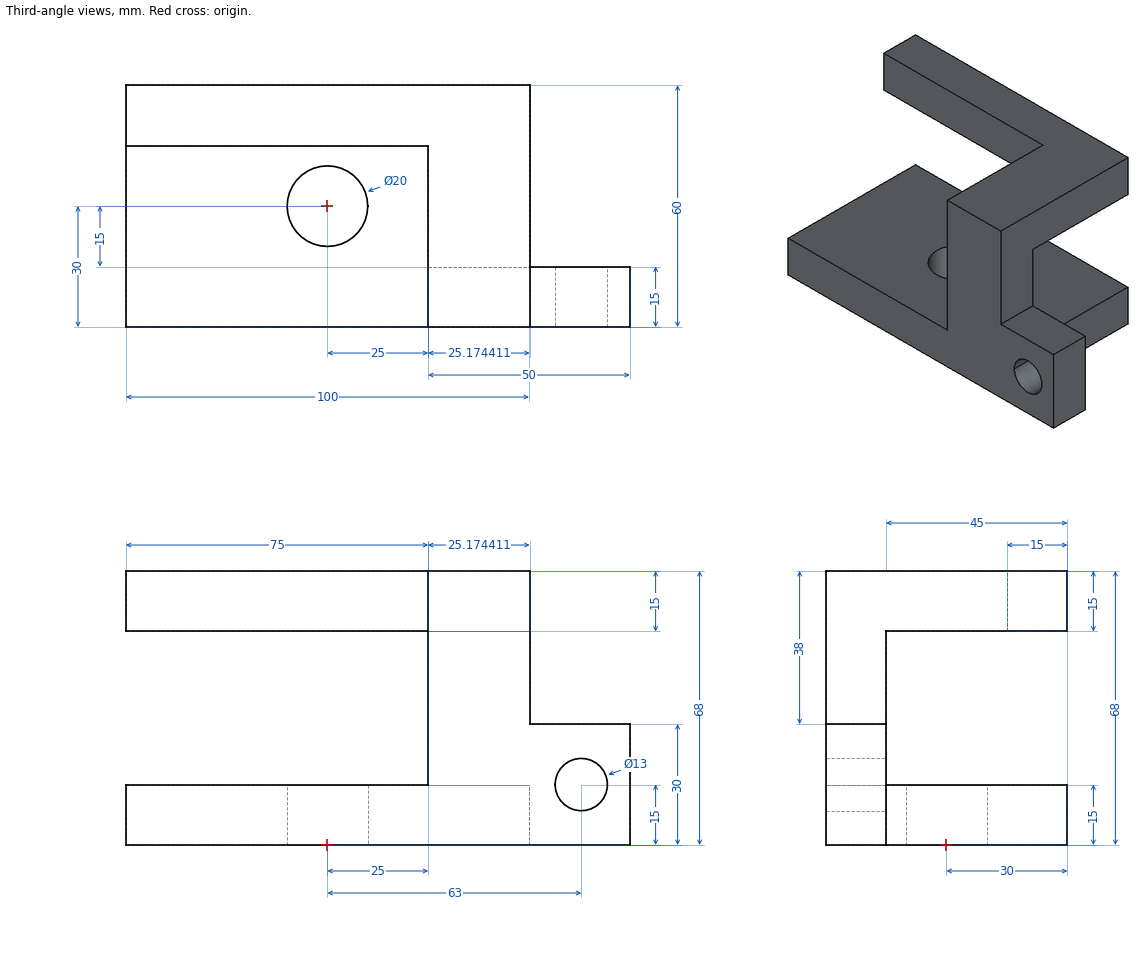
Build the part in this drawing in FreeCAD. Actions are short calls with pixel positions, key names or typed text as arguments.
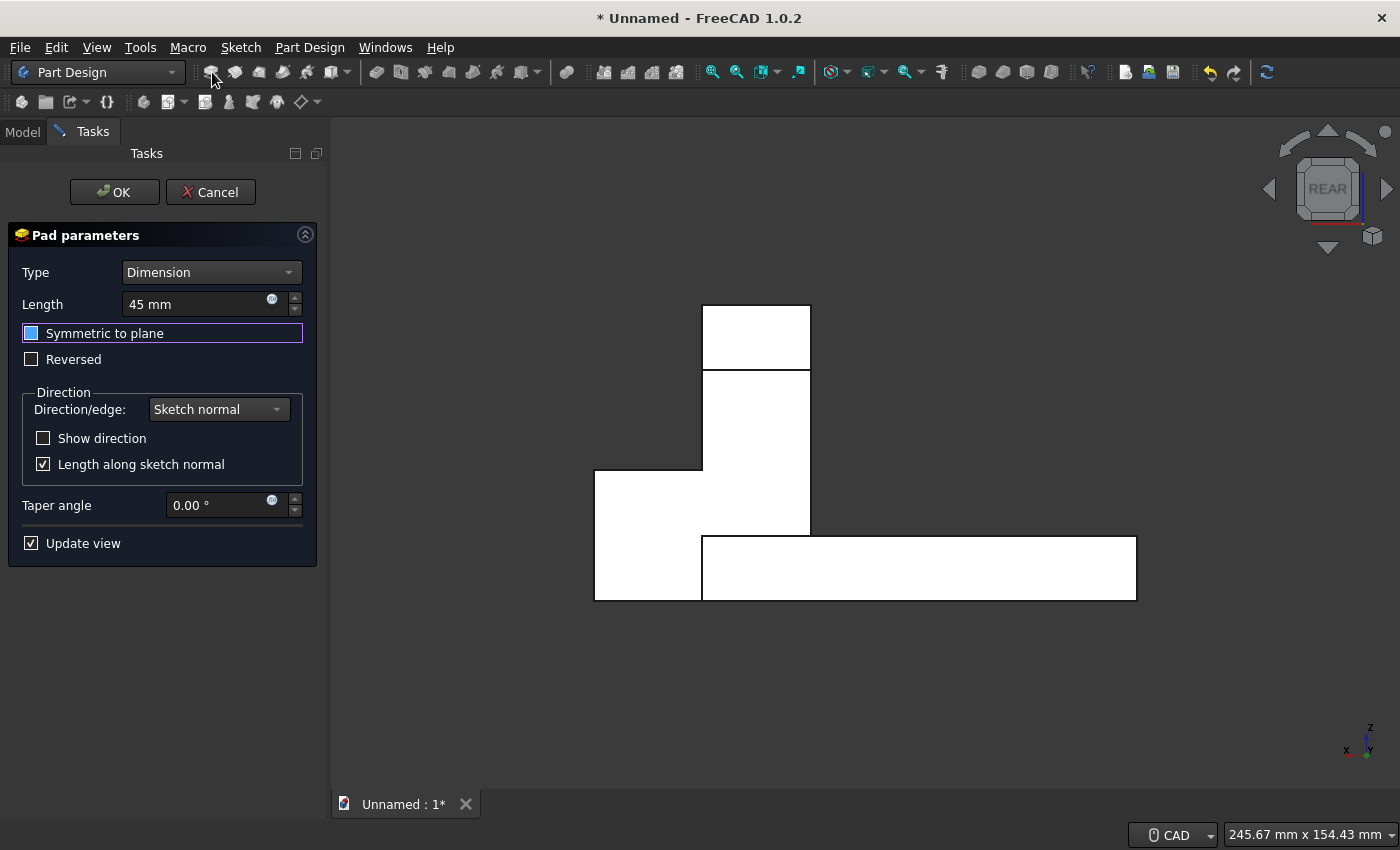
click(115, 192)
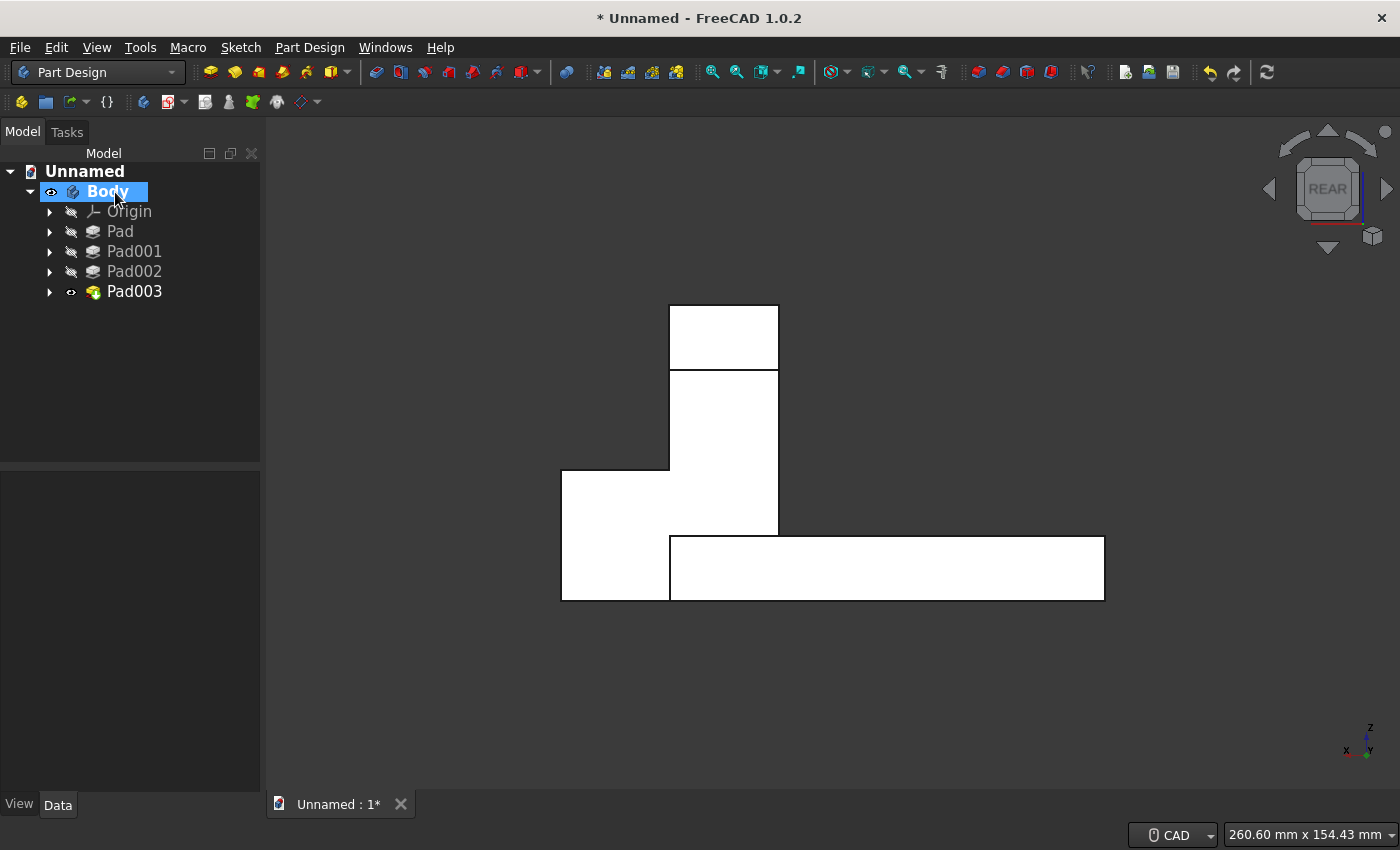
key(6)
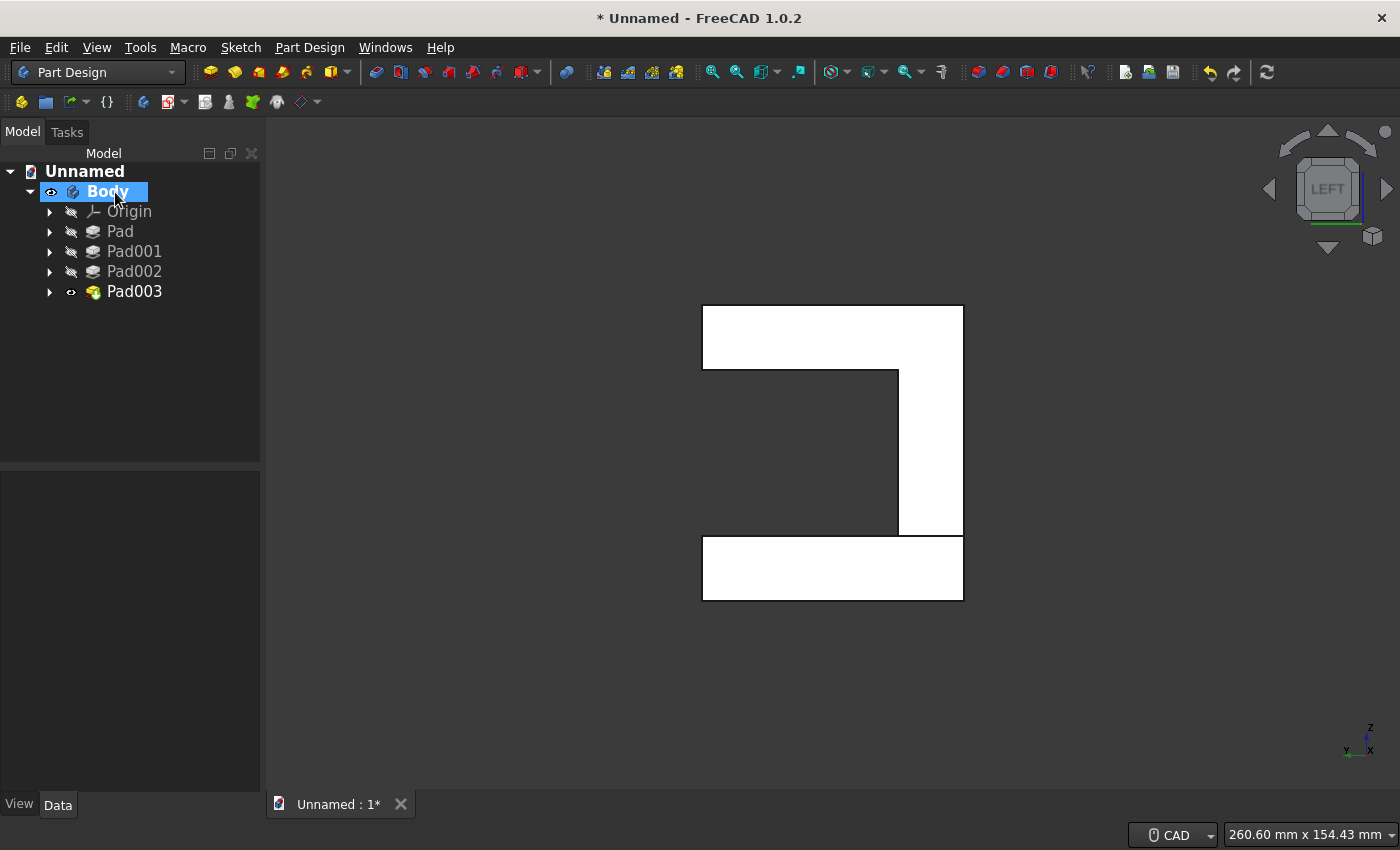
key(v)
key(f)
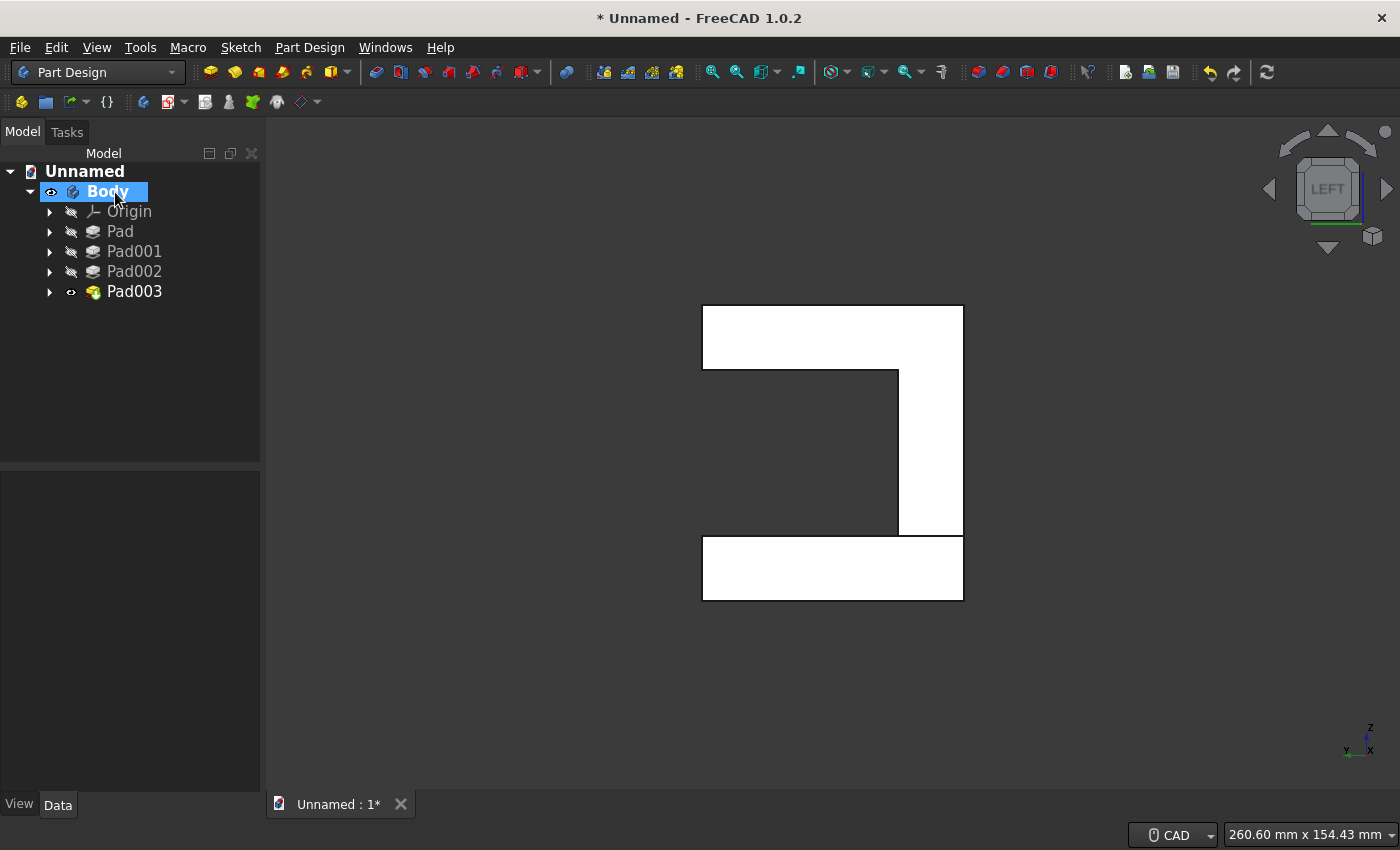
click(945, 353)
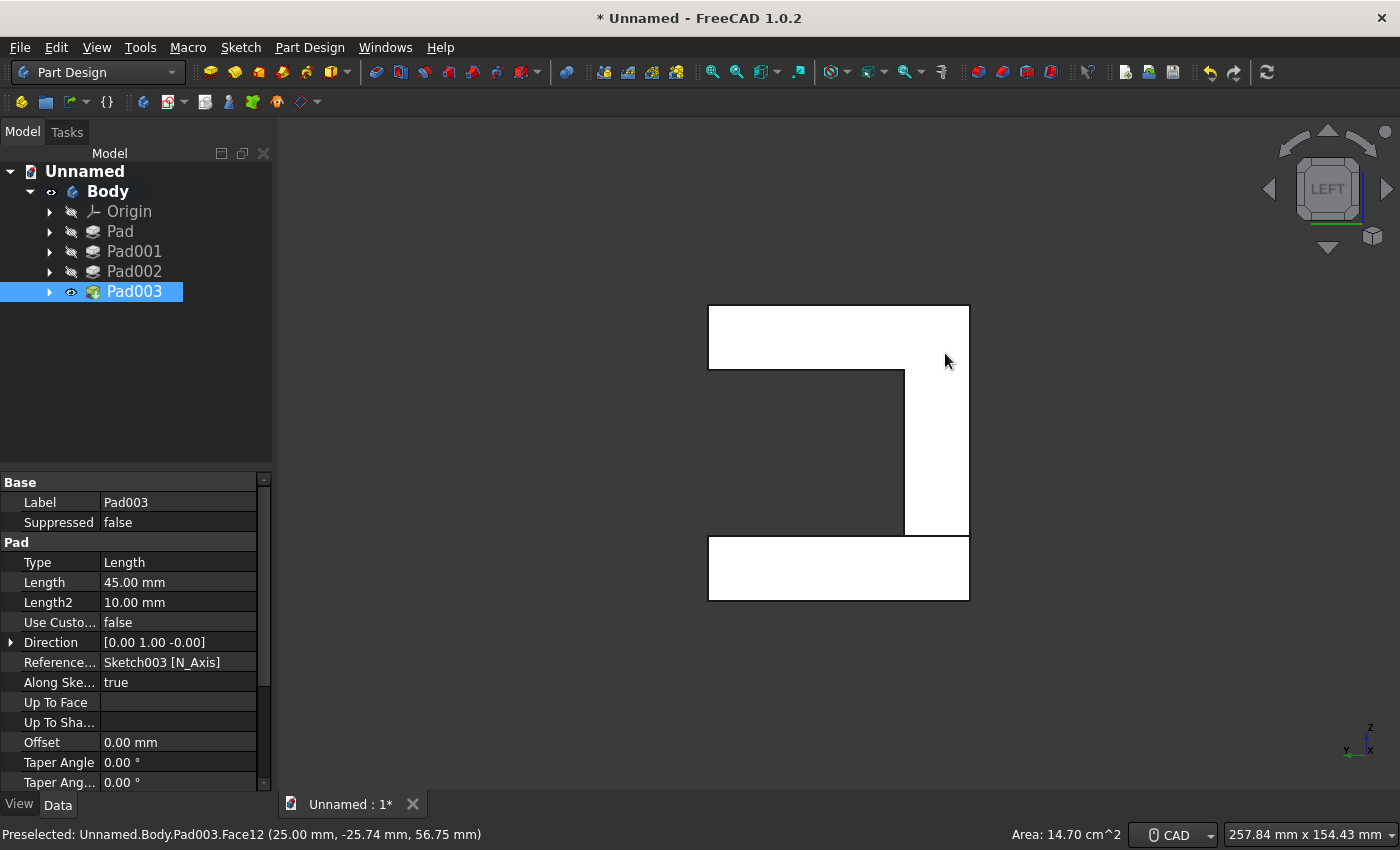
click(168, 102)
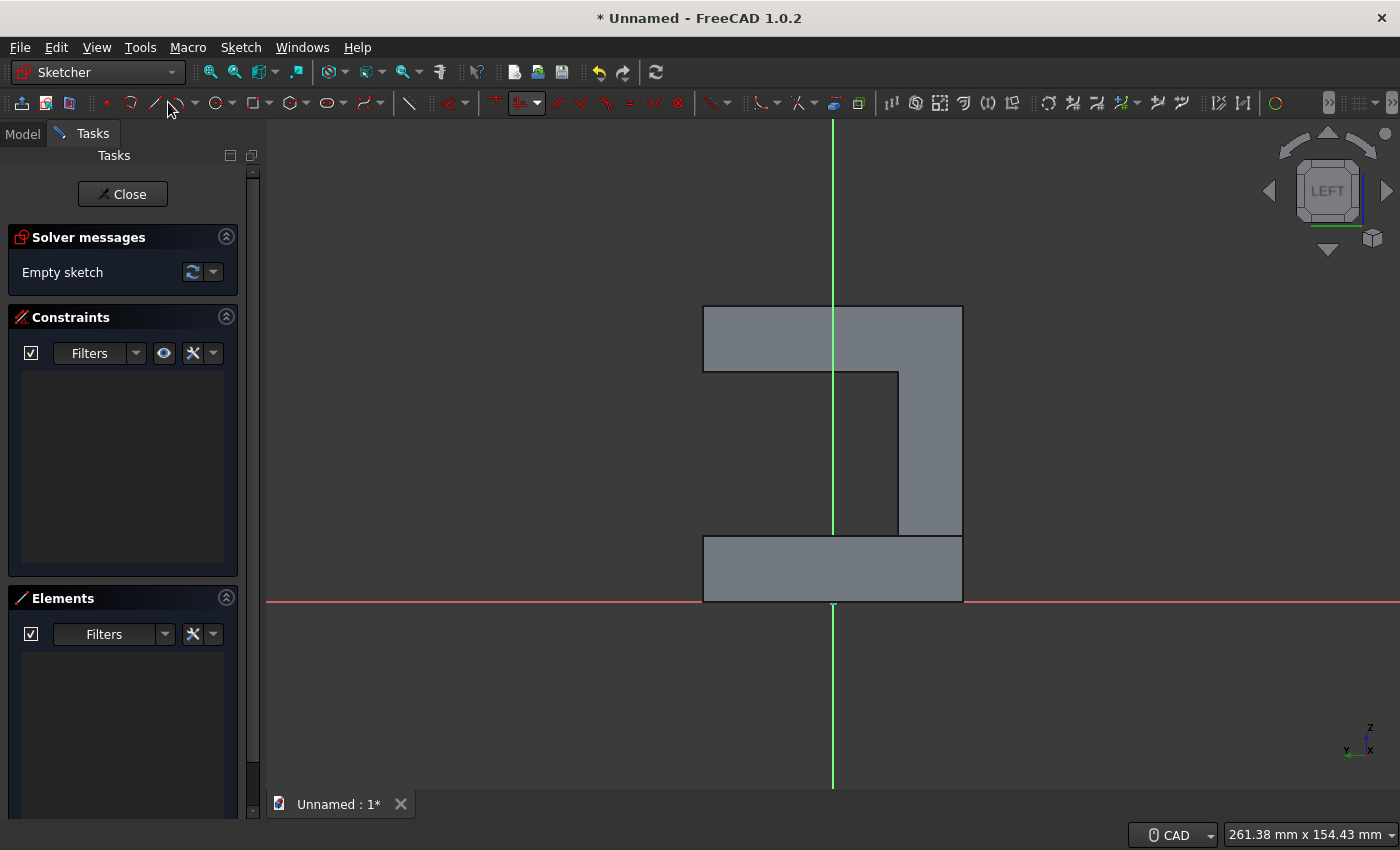
scroll(730, 316, up, 9)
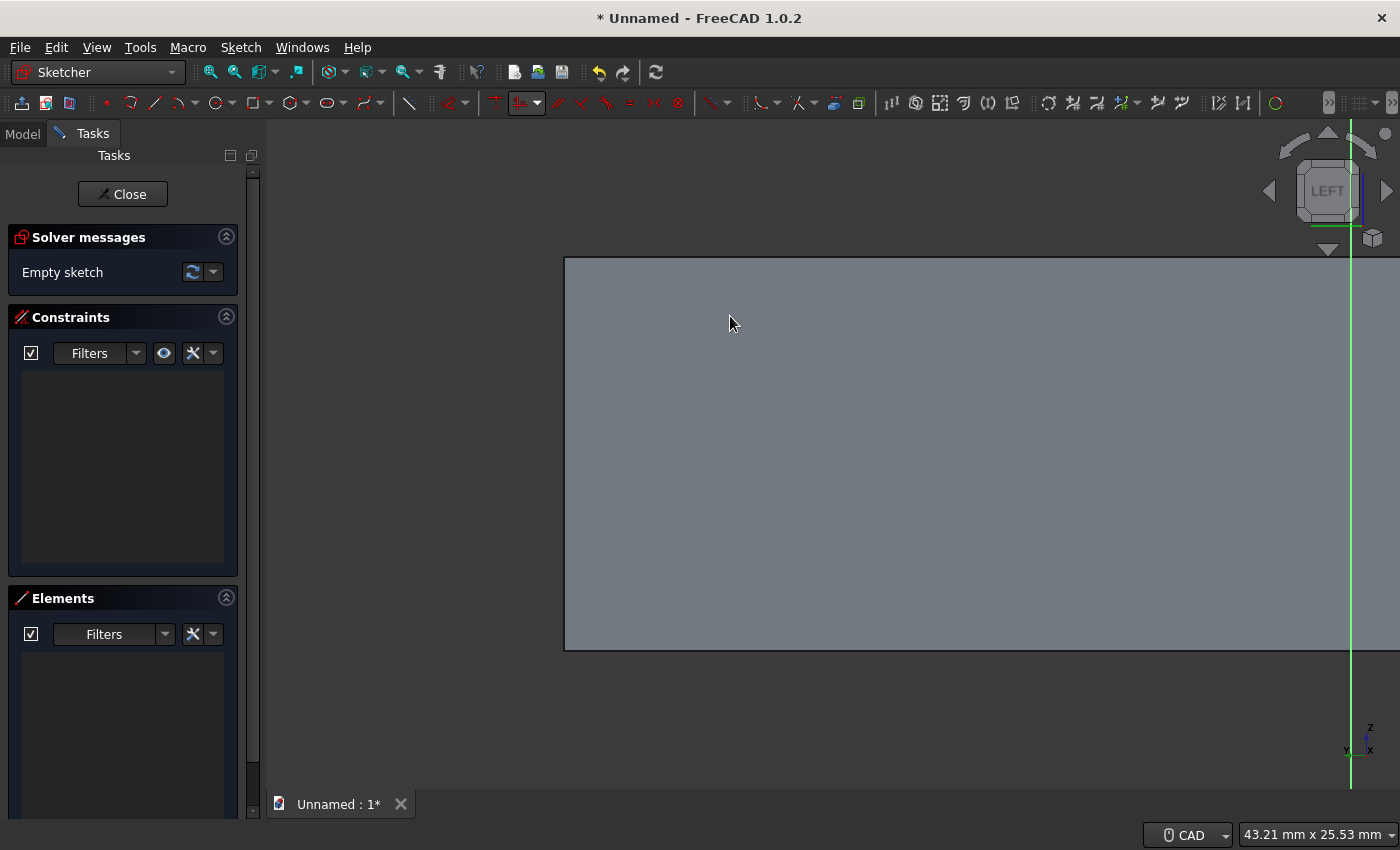
click(254, 104)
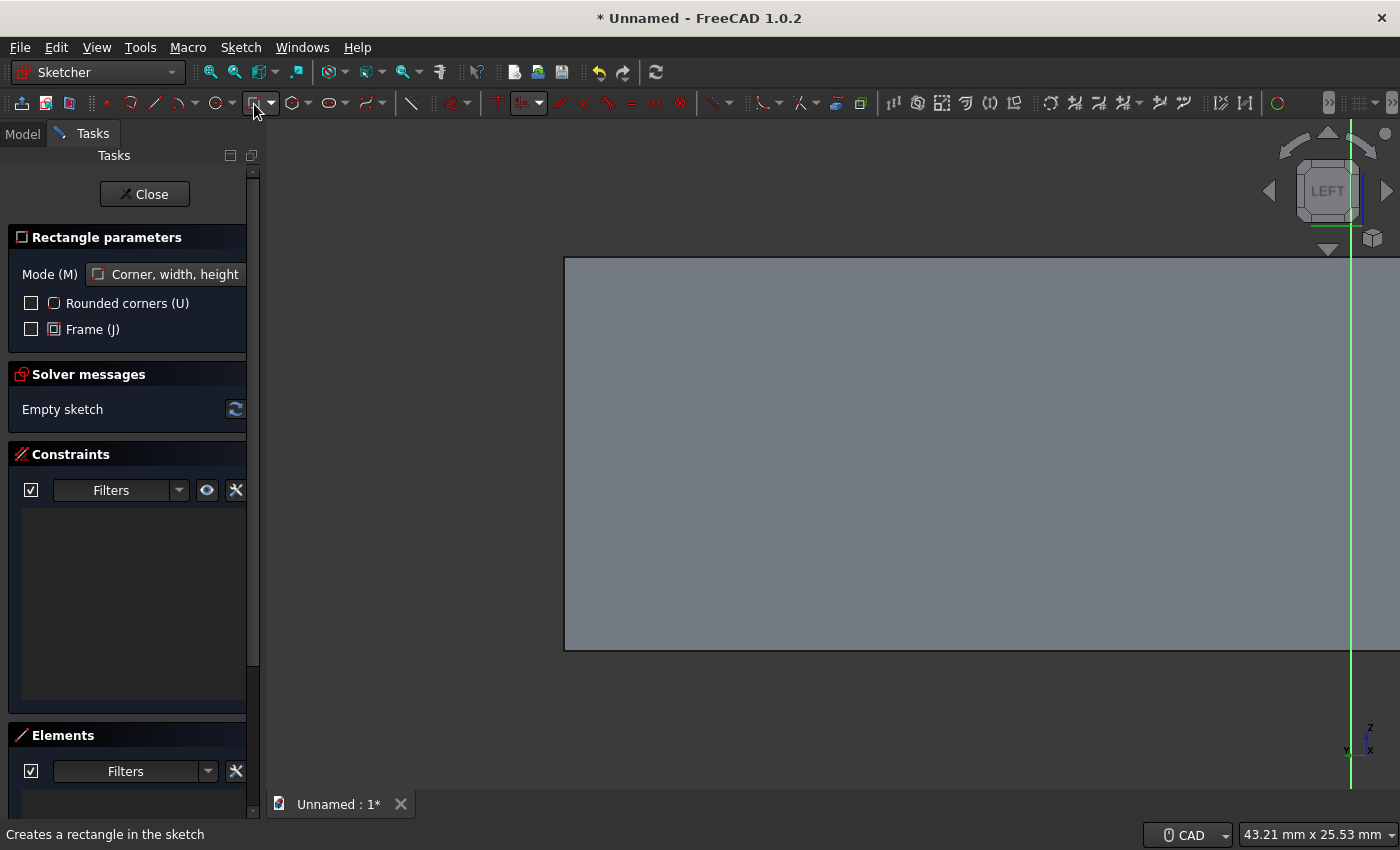
click(564, 257)
move(957, 651)